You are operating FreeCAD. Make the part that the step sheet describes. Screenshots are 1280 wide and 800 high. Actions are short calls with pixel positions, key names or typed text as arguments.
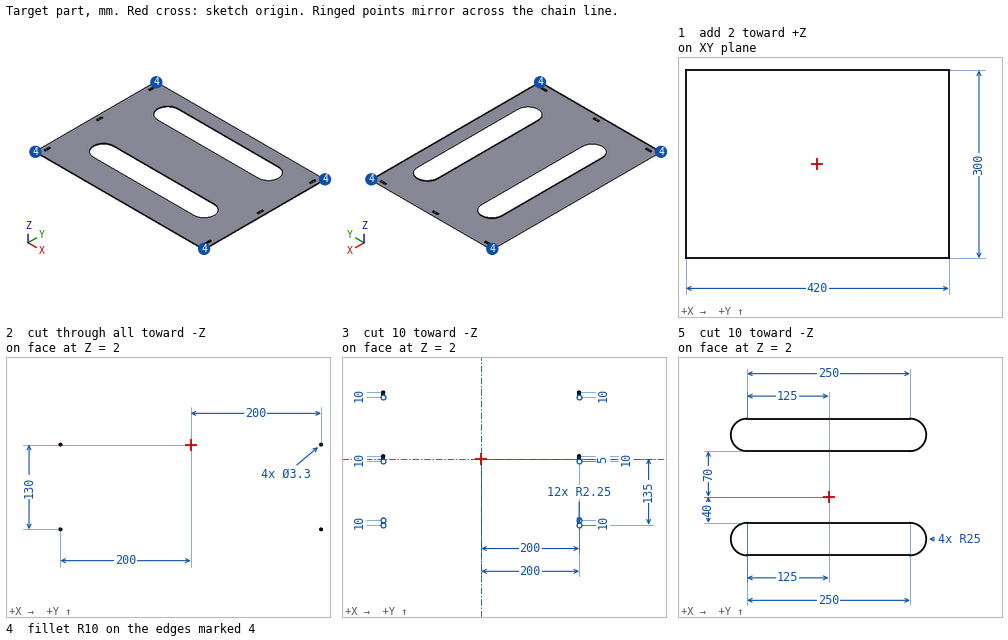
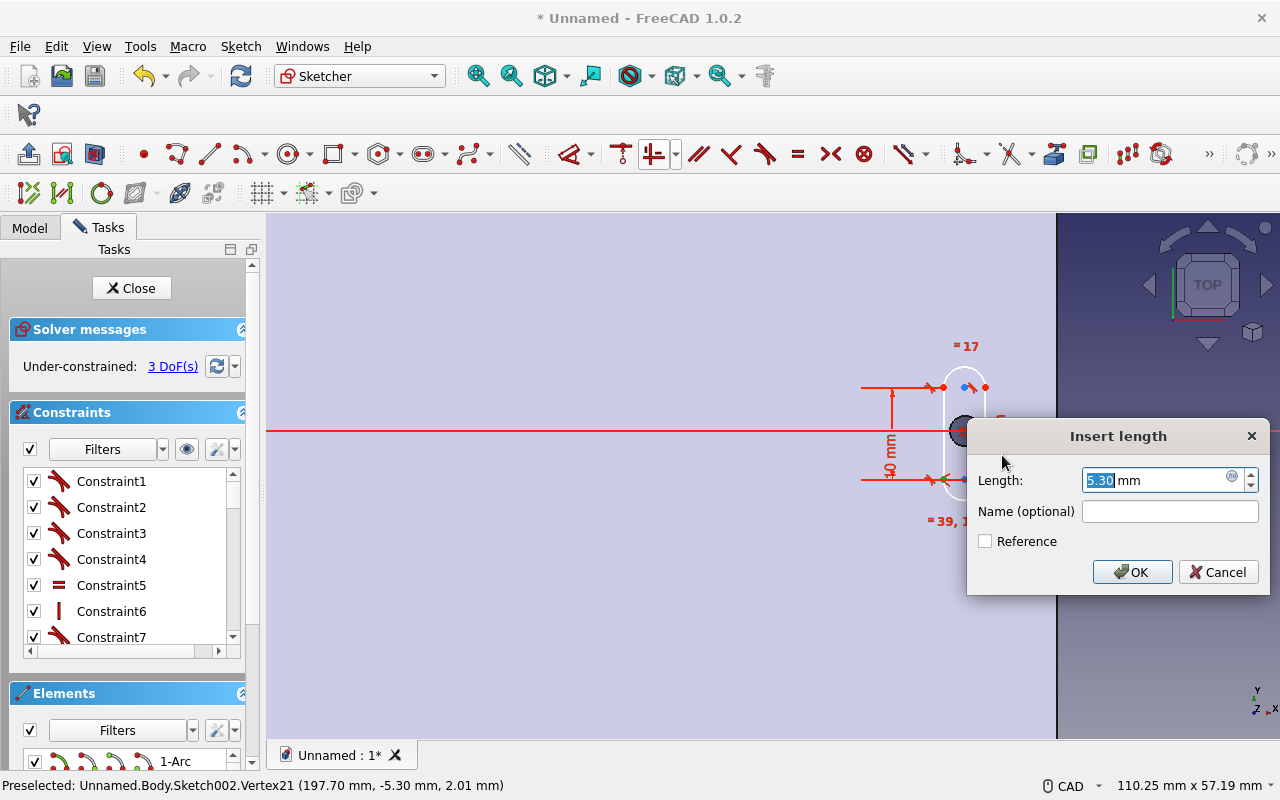
text(5)
key(Return)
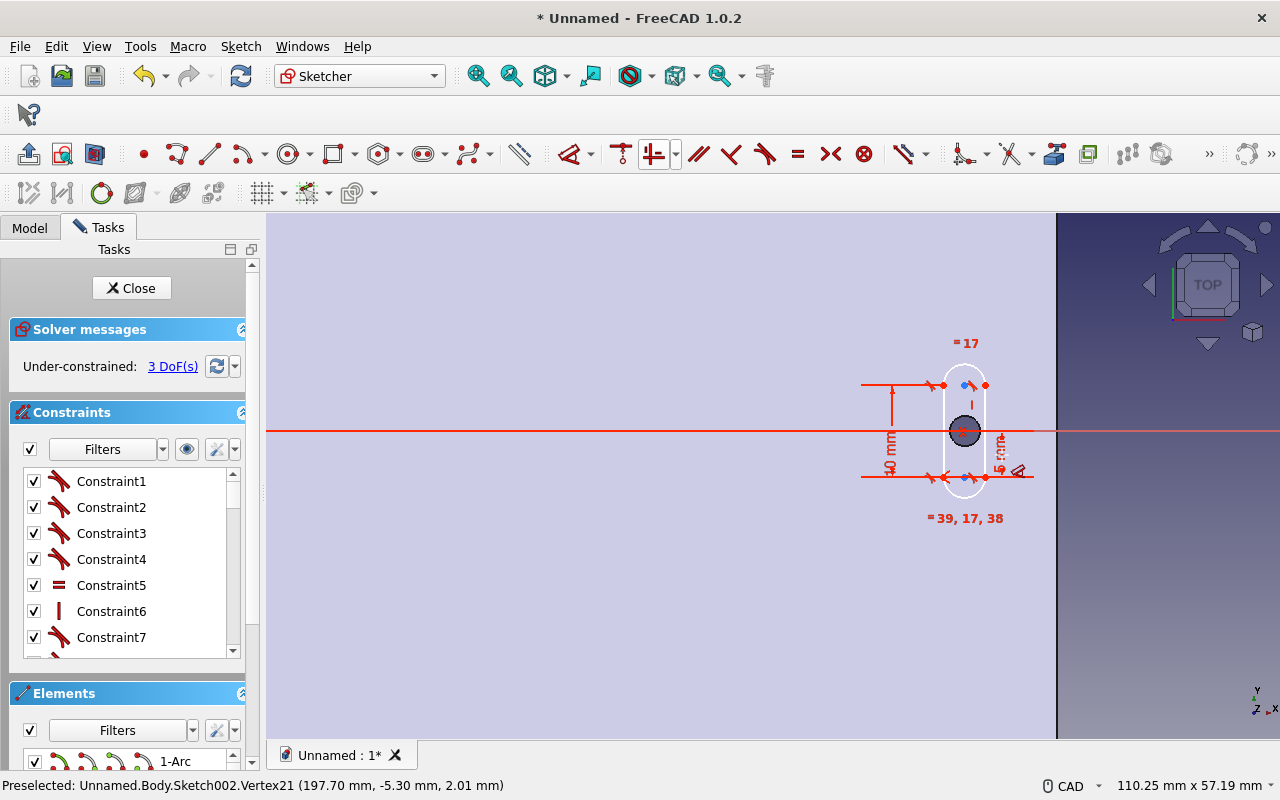
scroll(952, 483, down, 10)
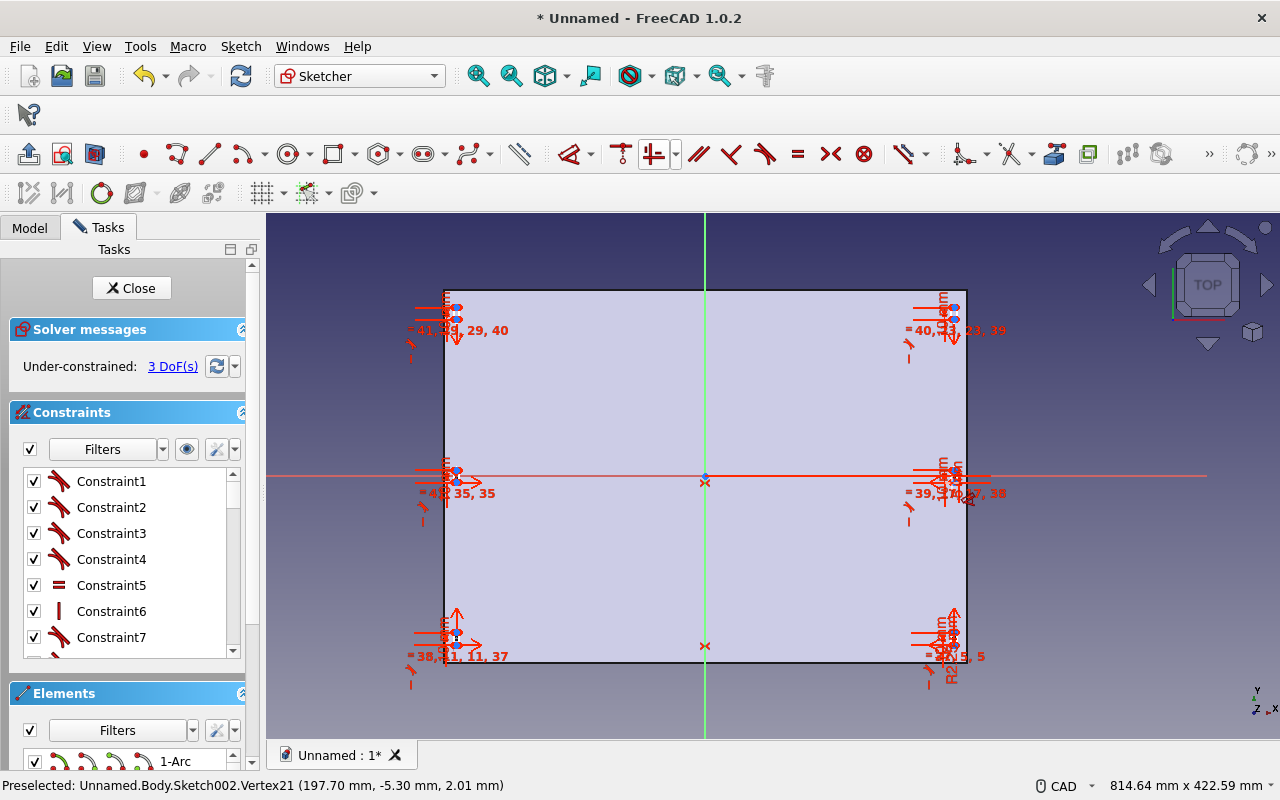
scroll(951, 645, up, 8)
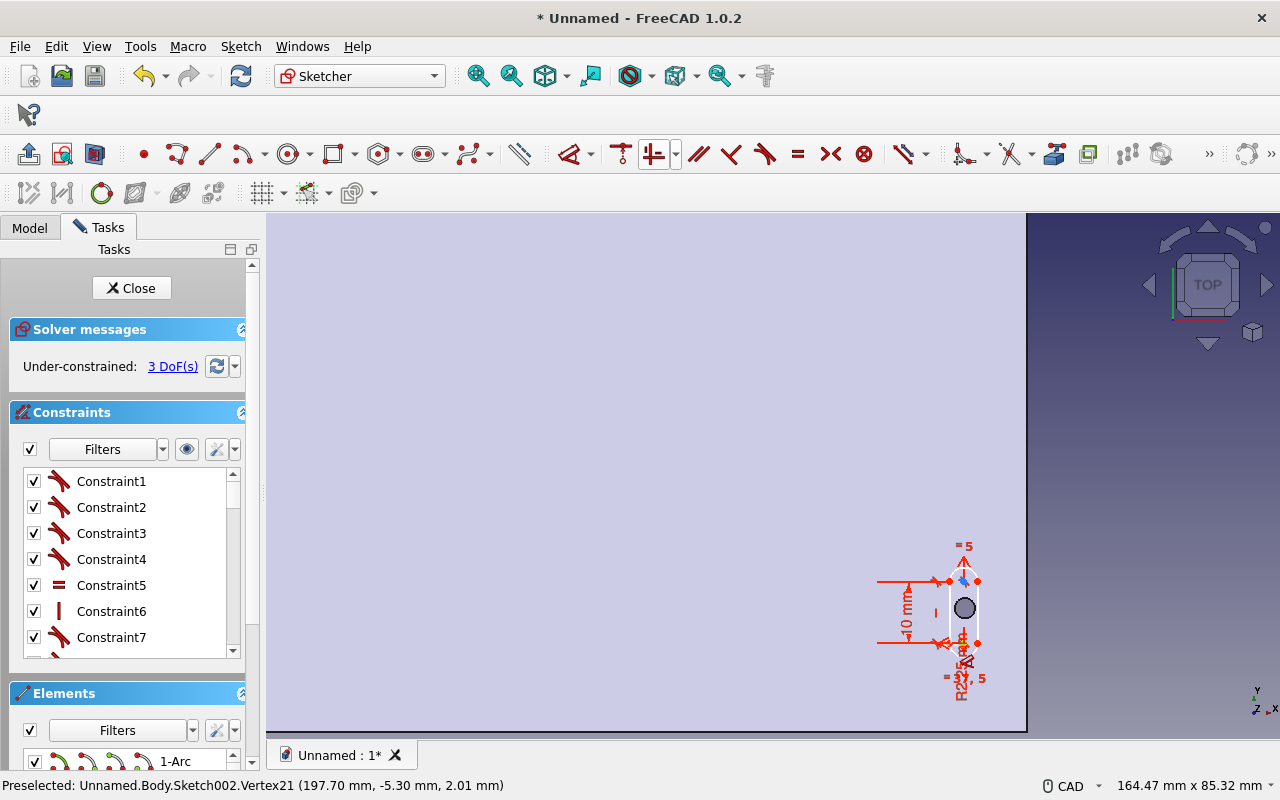
click(950, 643)
click(984, 442)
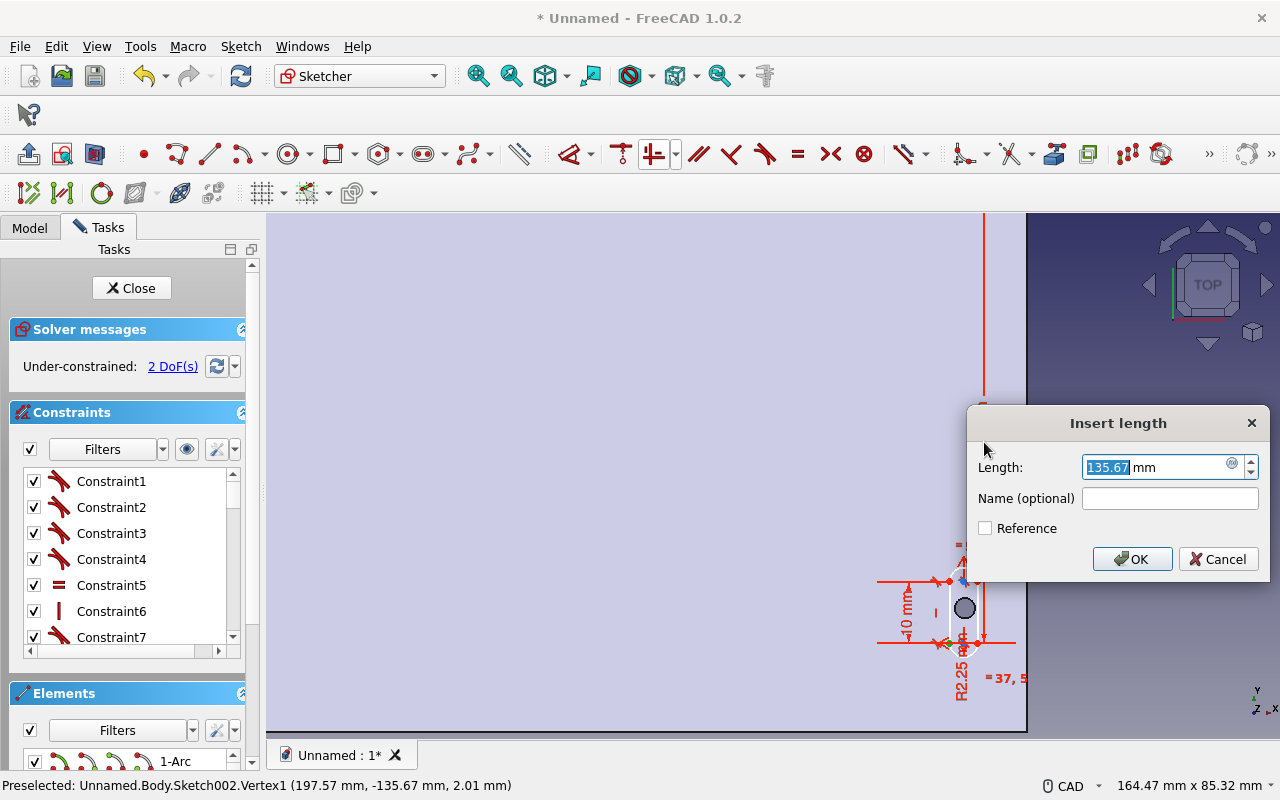
text(135)
key(Return)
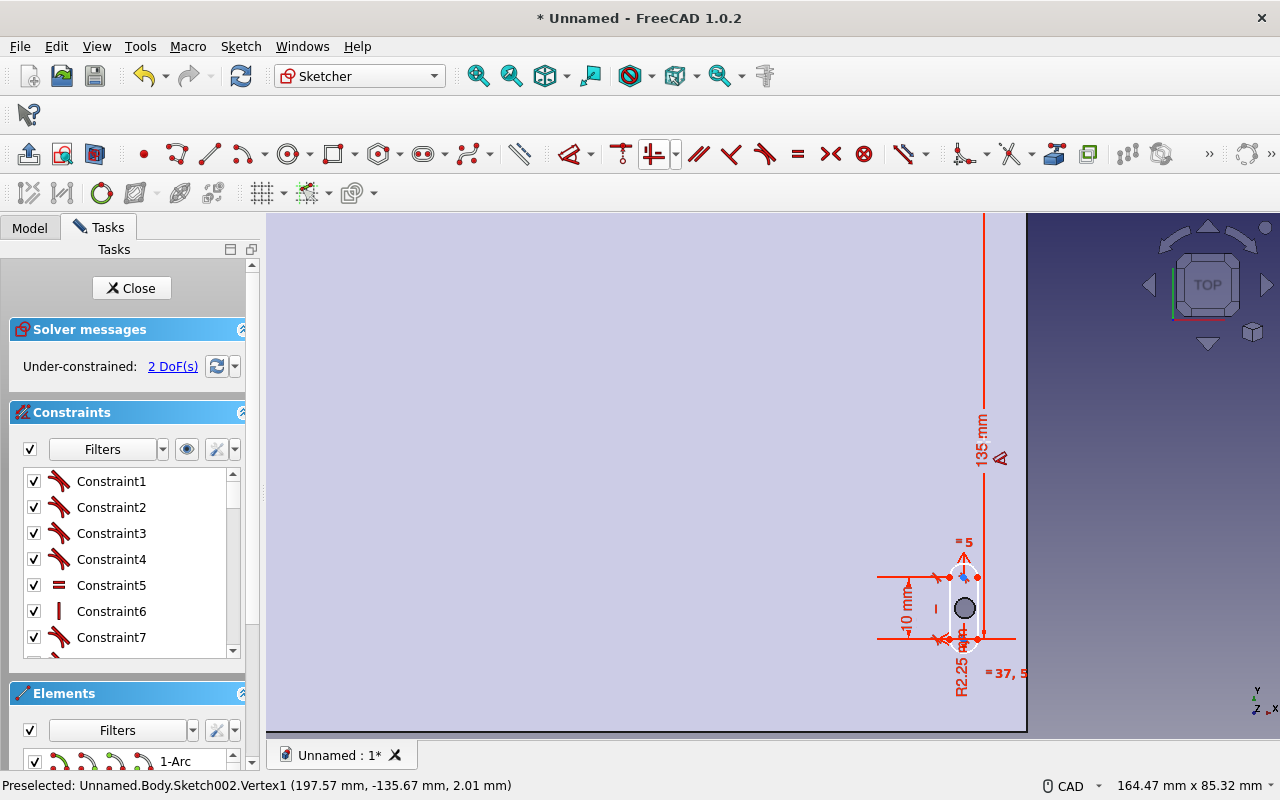
click(964, 639)
click(629, 673)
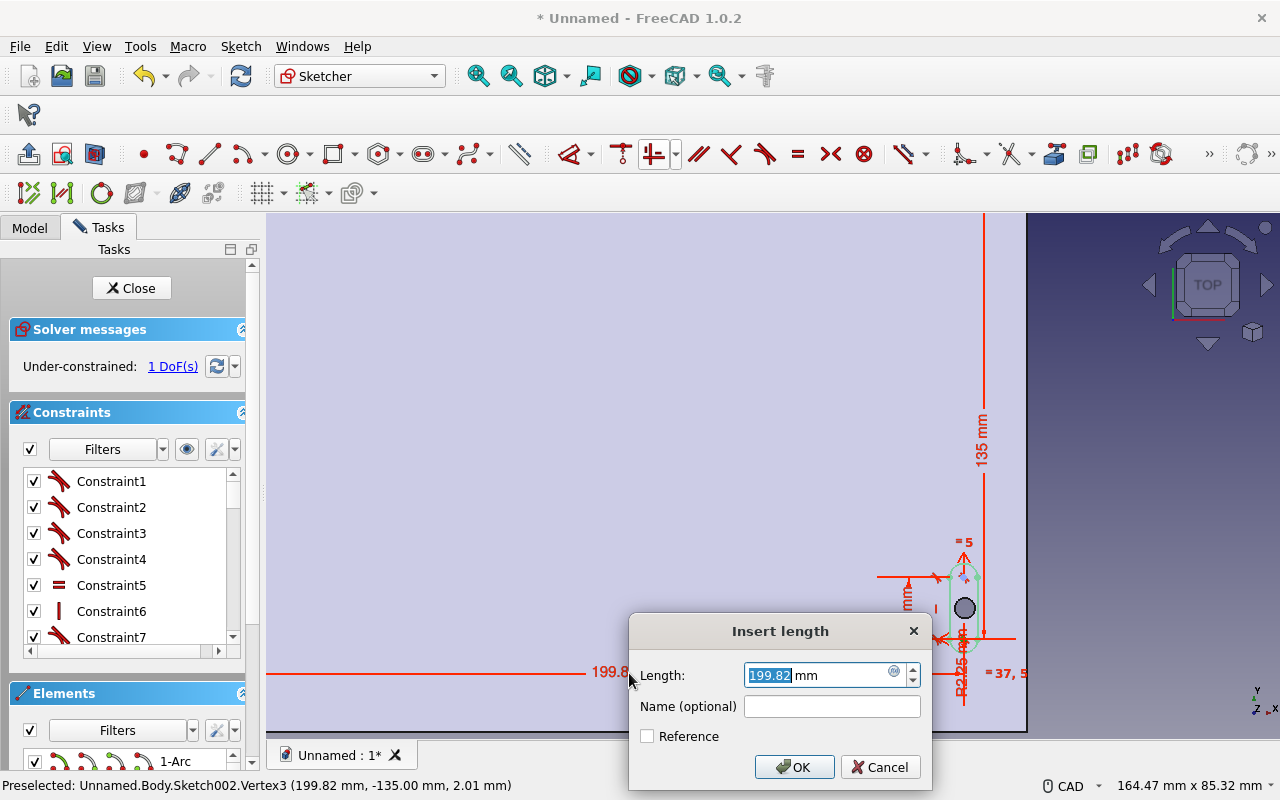
text(200)
key(Return)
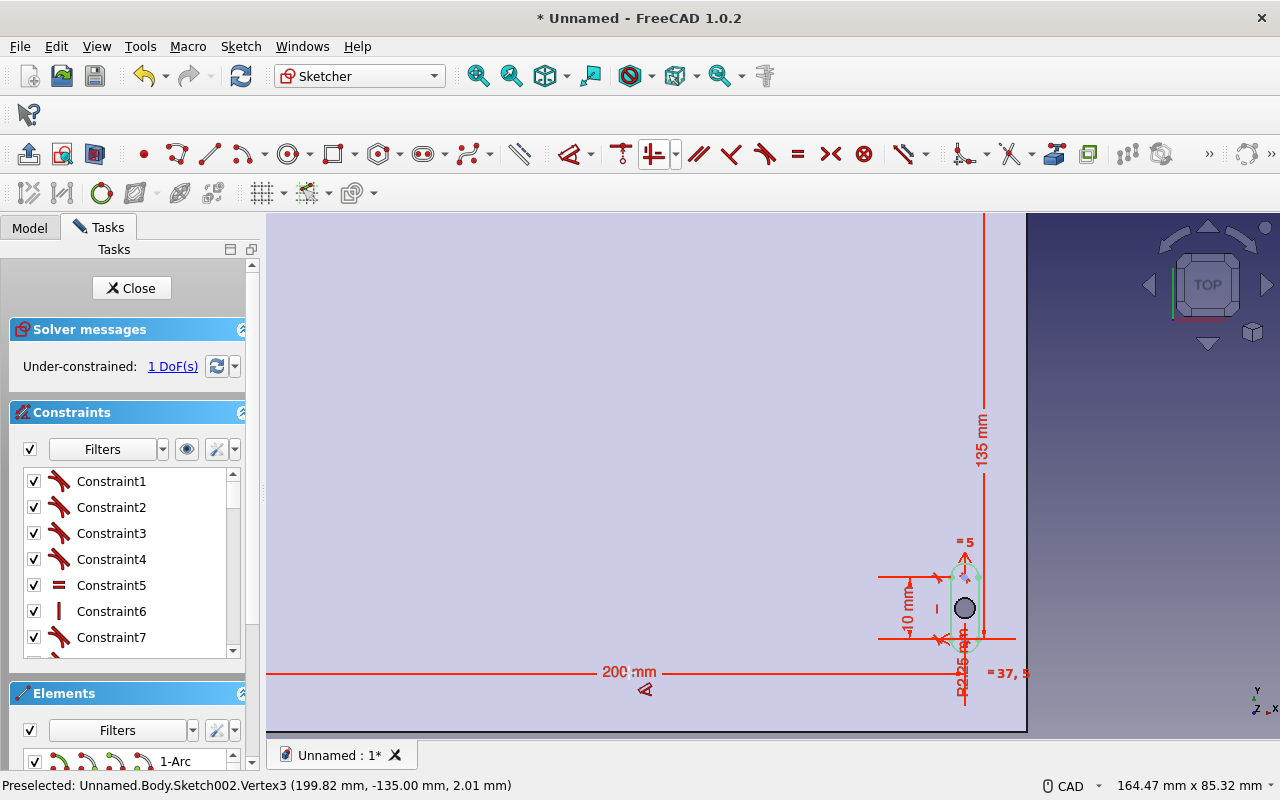
scroll(951, 645, down, 8)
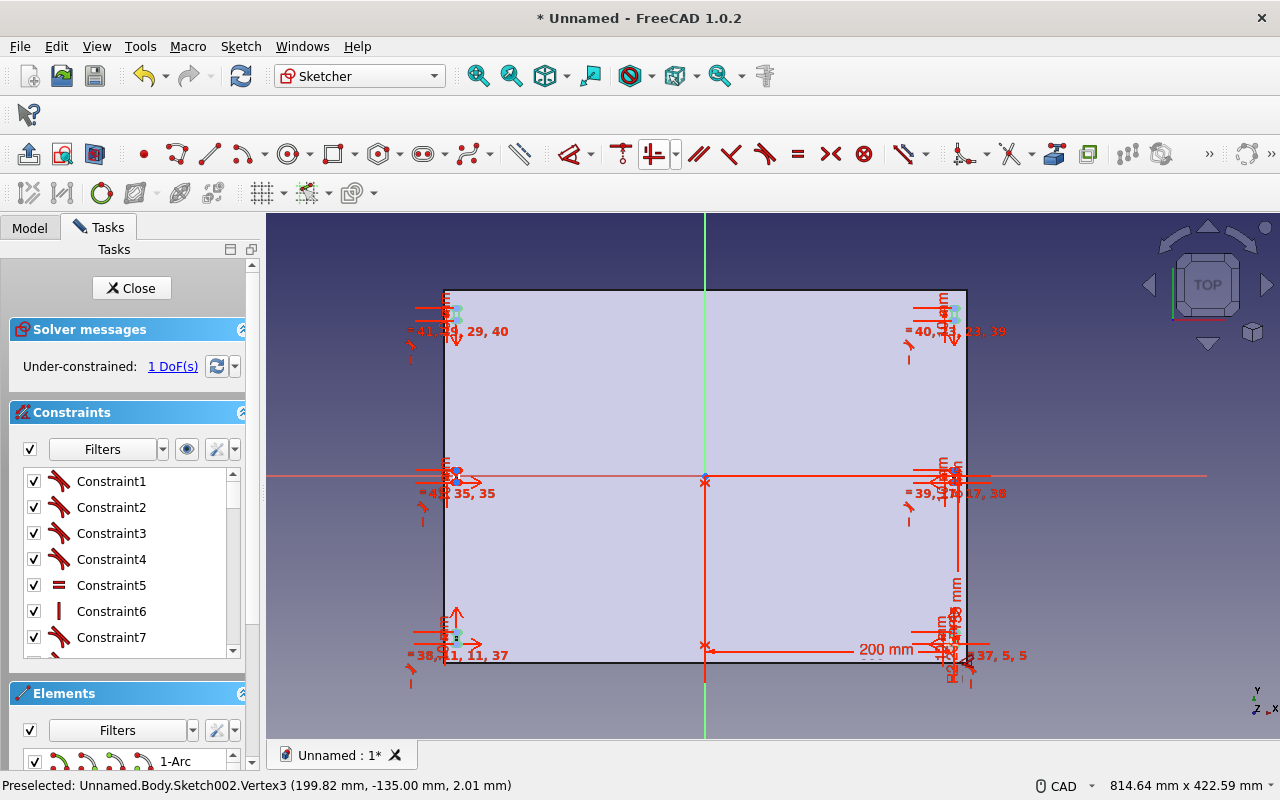
scroll(954, 483, up, 8)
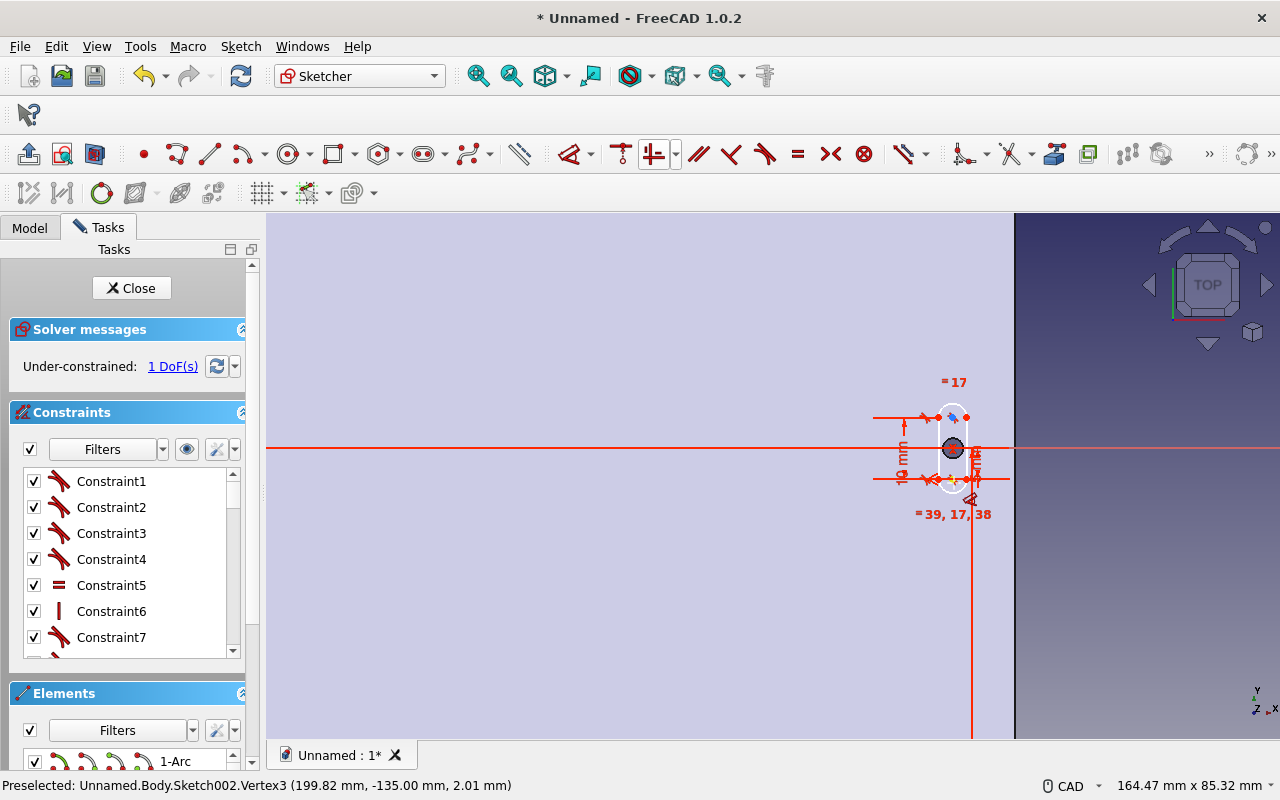
click(953, 479)
click(623, 513)